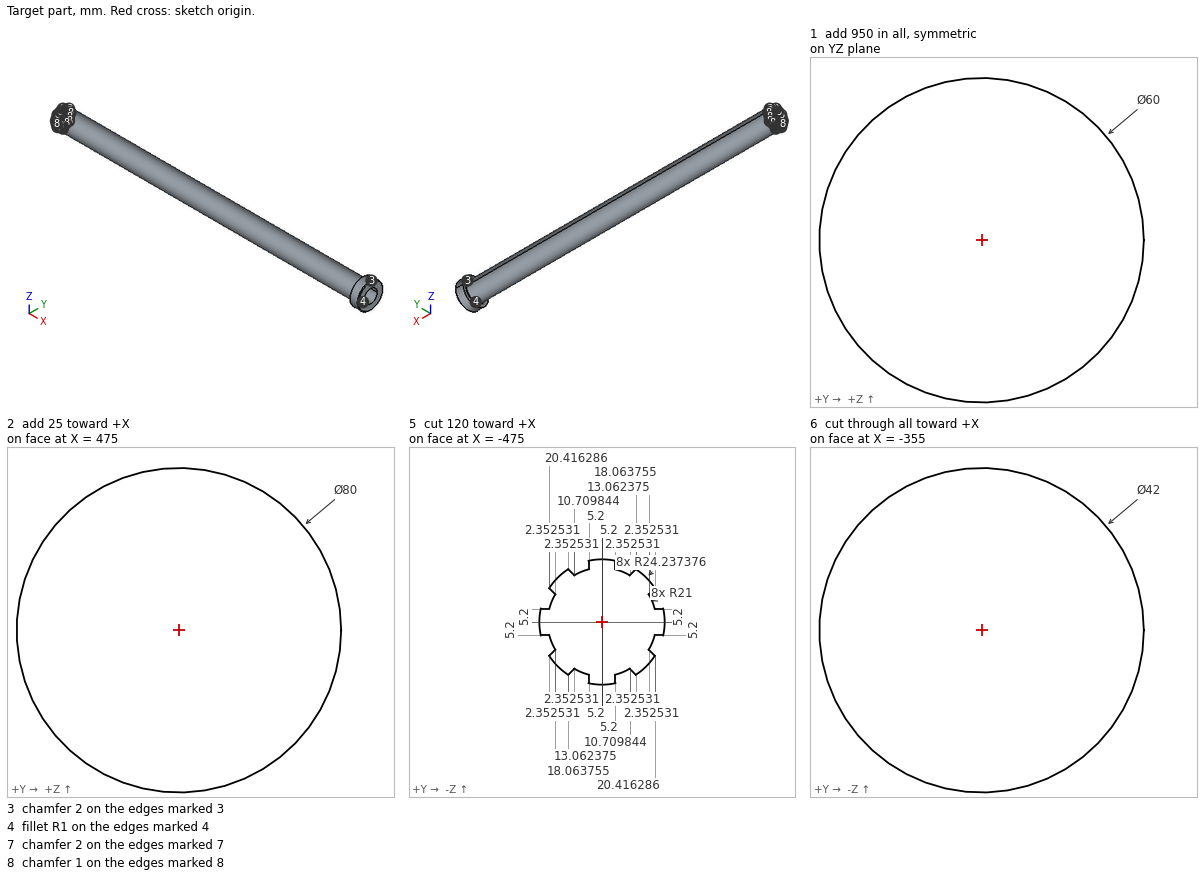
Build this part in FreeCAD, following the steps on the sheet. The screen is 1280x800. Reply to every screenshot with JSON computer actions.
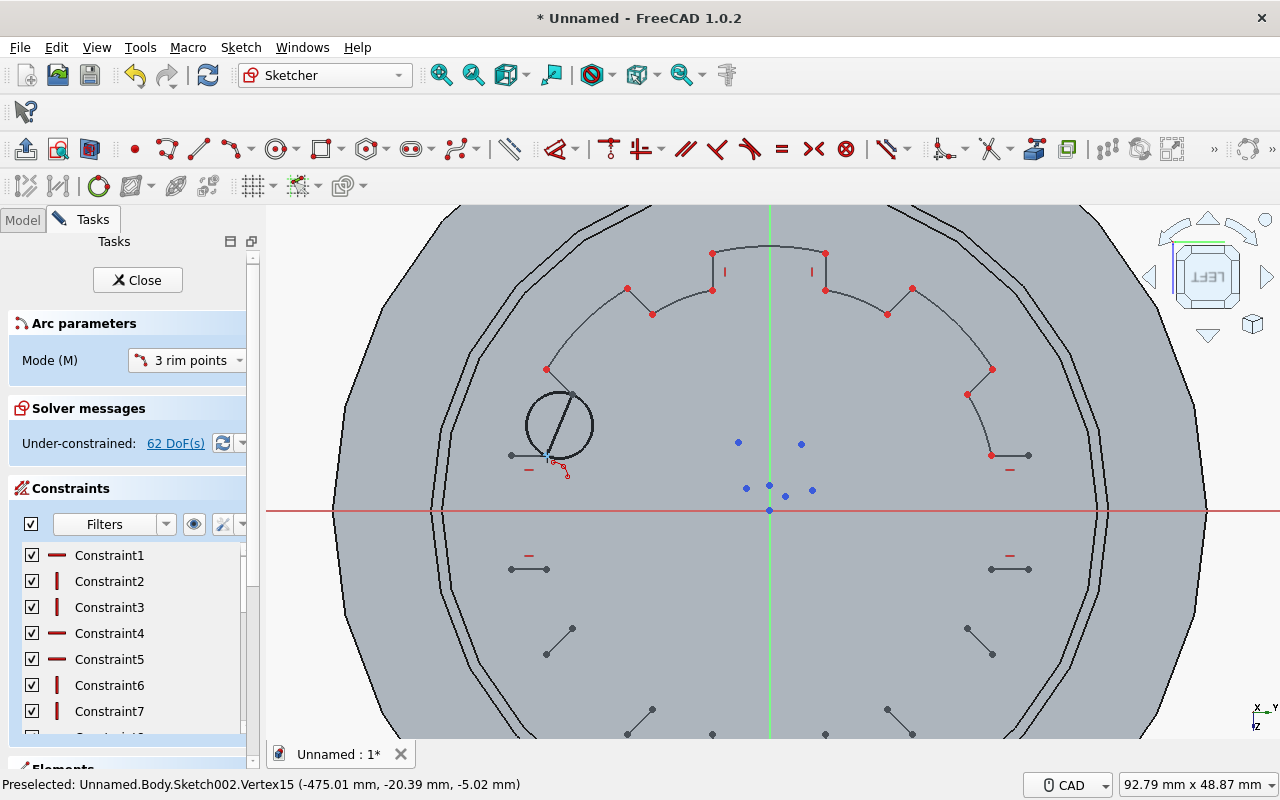
{"action": "scroll", "coordinate": [558, 423], "scroll_direction": "up", "scroll_amount": 10}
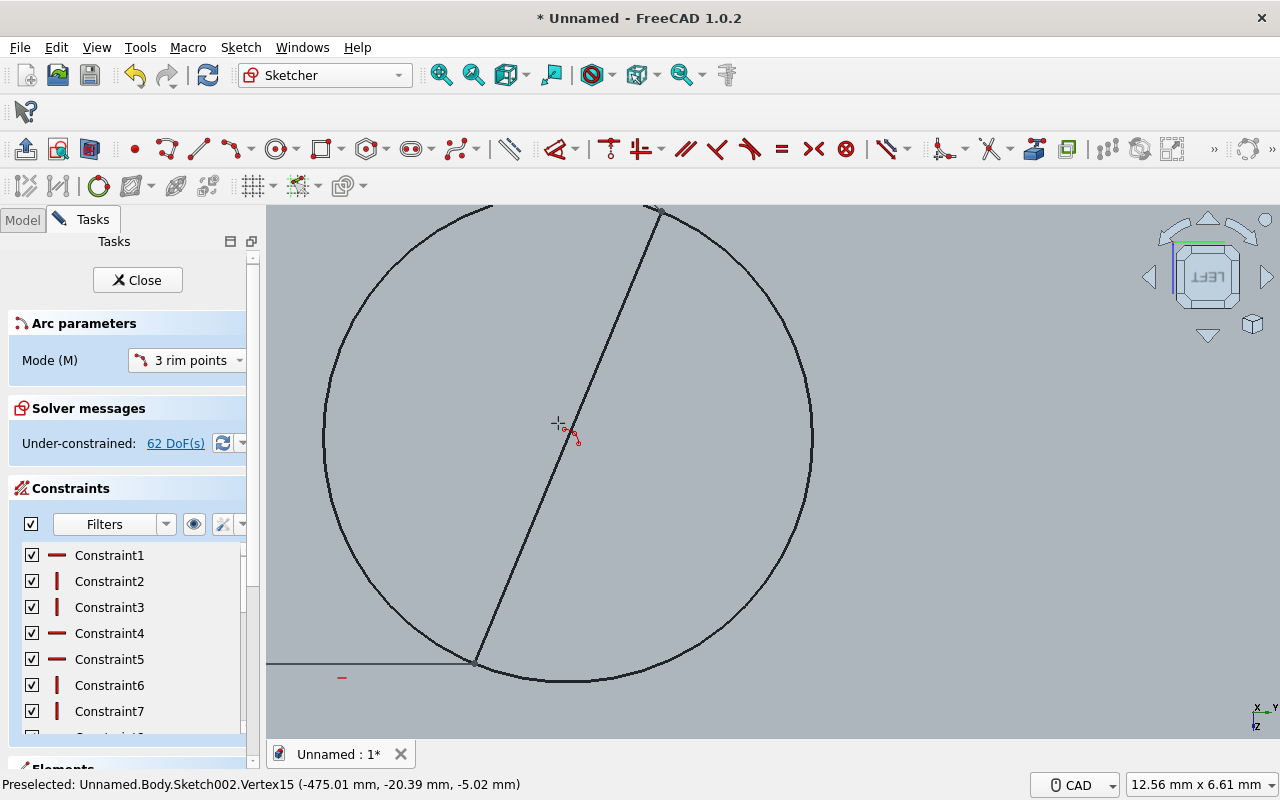
{"action": "left_click", "coordinate": [554, 420]}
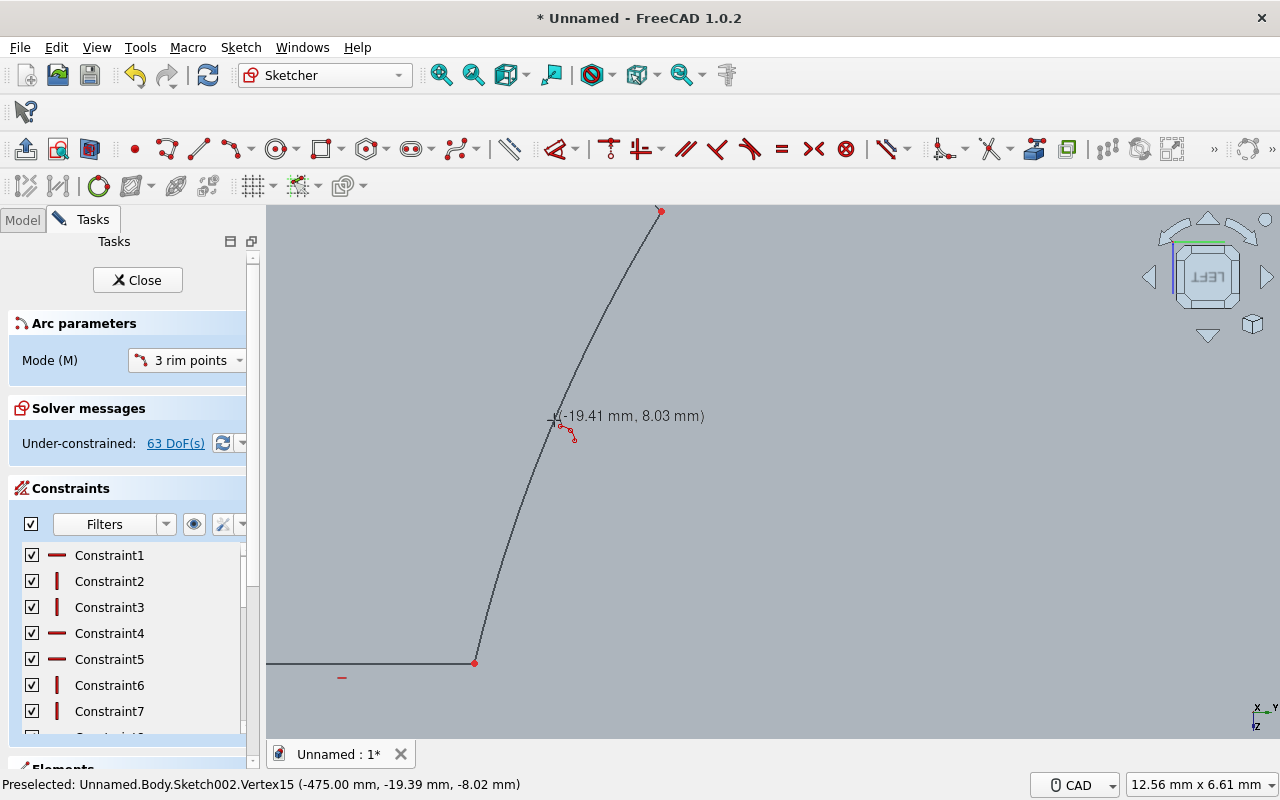
{"action": "scroll", "coordinate": [563, 412], "scroll_direction": "down", "scroll_amount": 12}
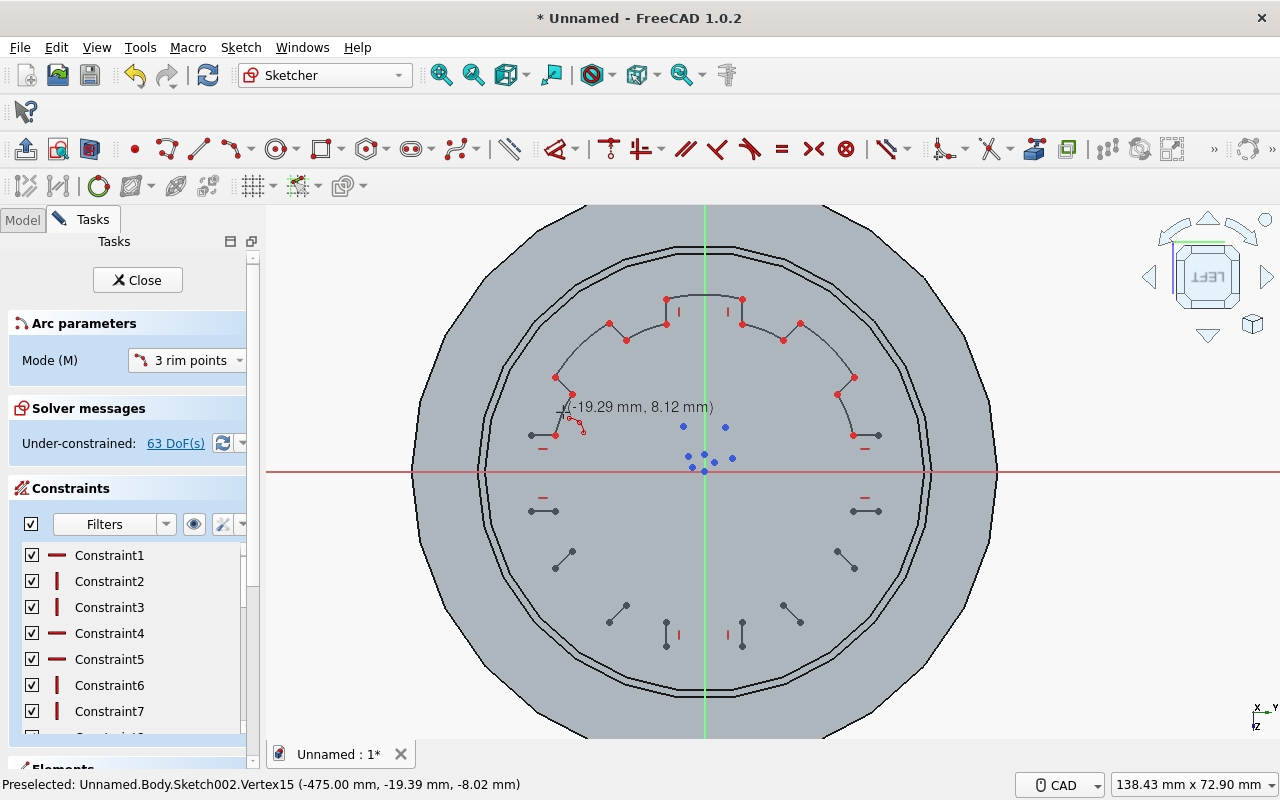
{"action": "scroll", "coordinate": [531, 434], "scroll_direction": "up", "scroll_amount": 2}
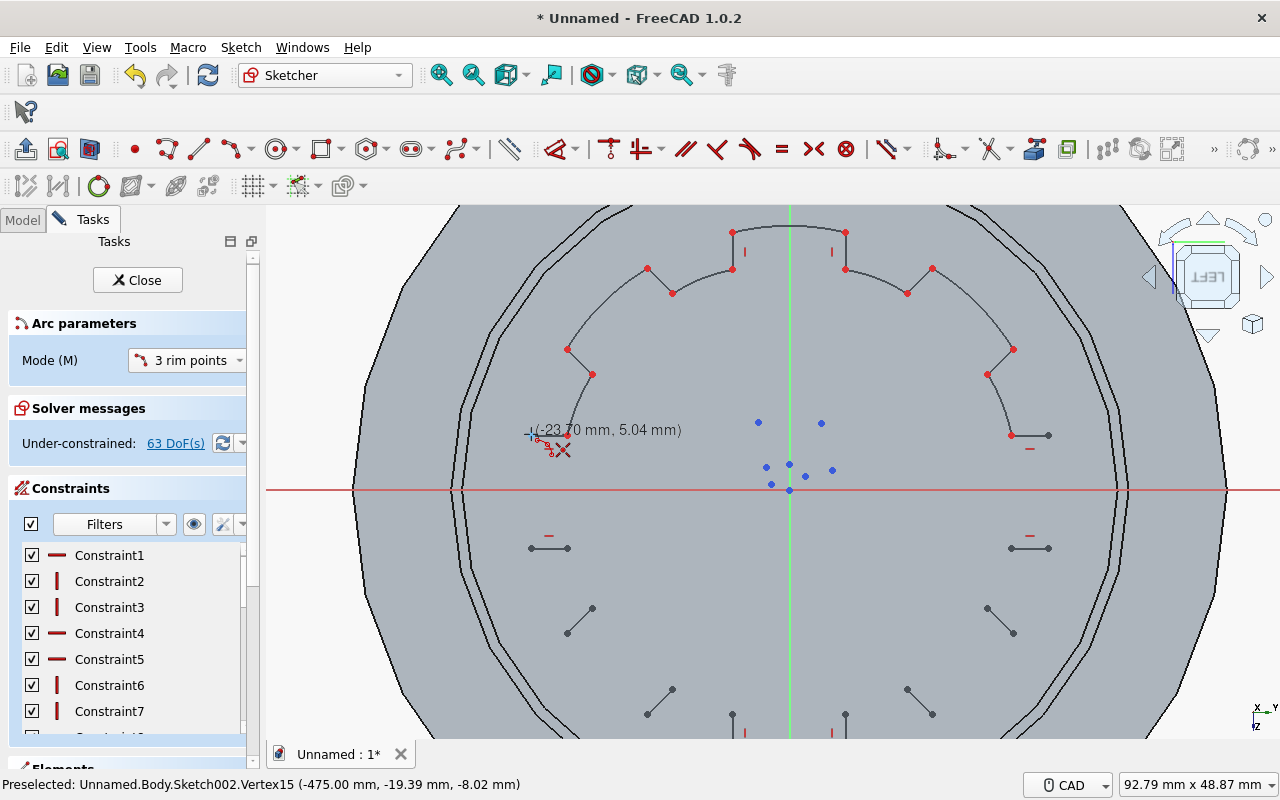
{"action": "left_click", "coordinate": [531, 436]}
{"action": "left_click", "coordinate": [531, 549]}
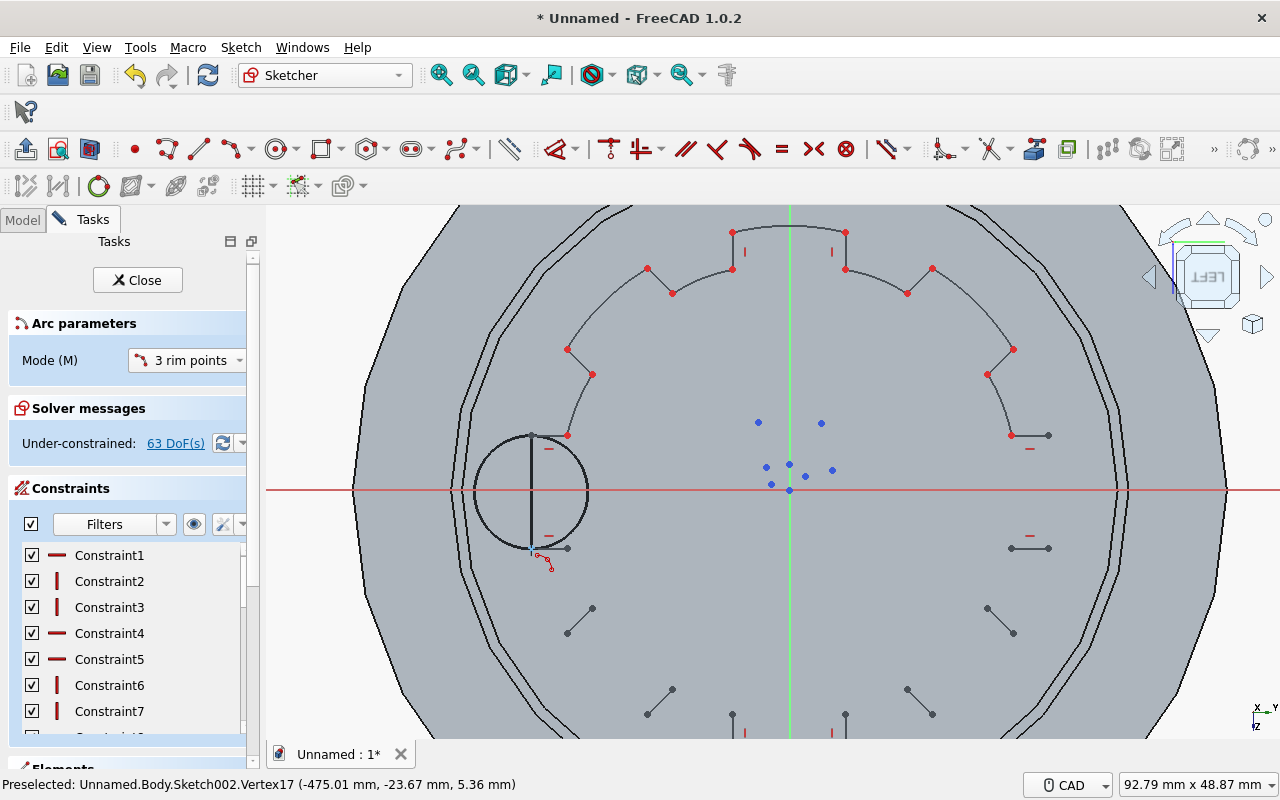
{"action": "scroll", "coordinate": [525, 479], "scroll_direction": "up", "scroll_amount": 5}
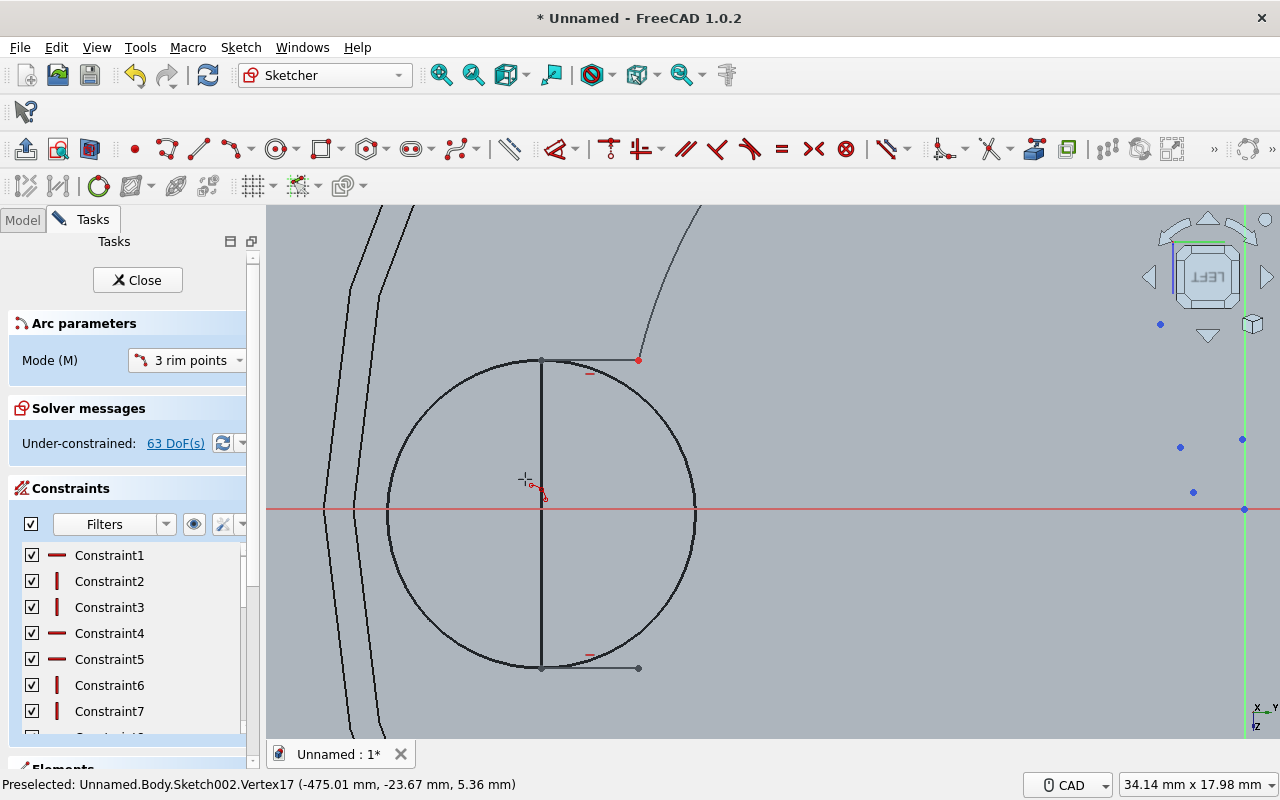
{"action": "left_click", "coordinate": [525, 478]}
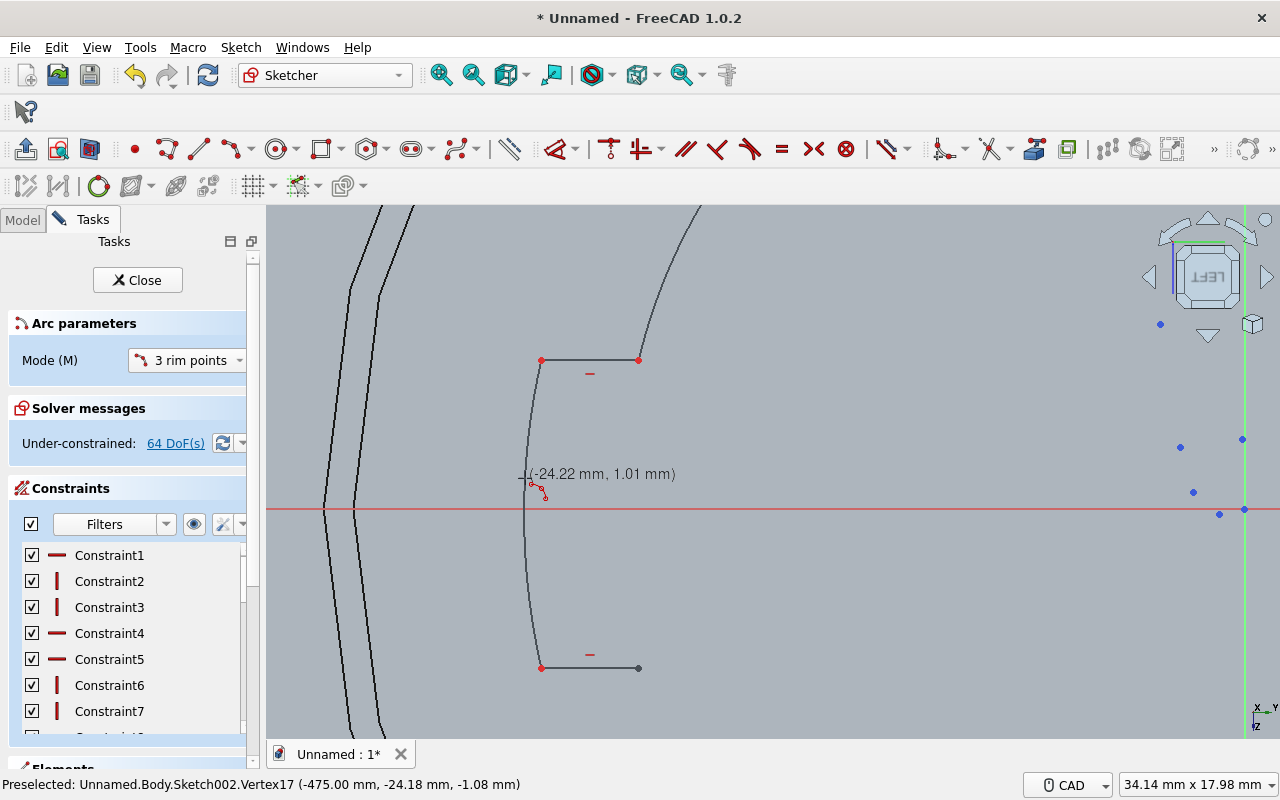
{"action": "scroll", "coordinate": [528, 460], "scroll_direction": "down", "scroll_amount": 7}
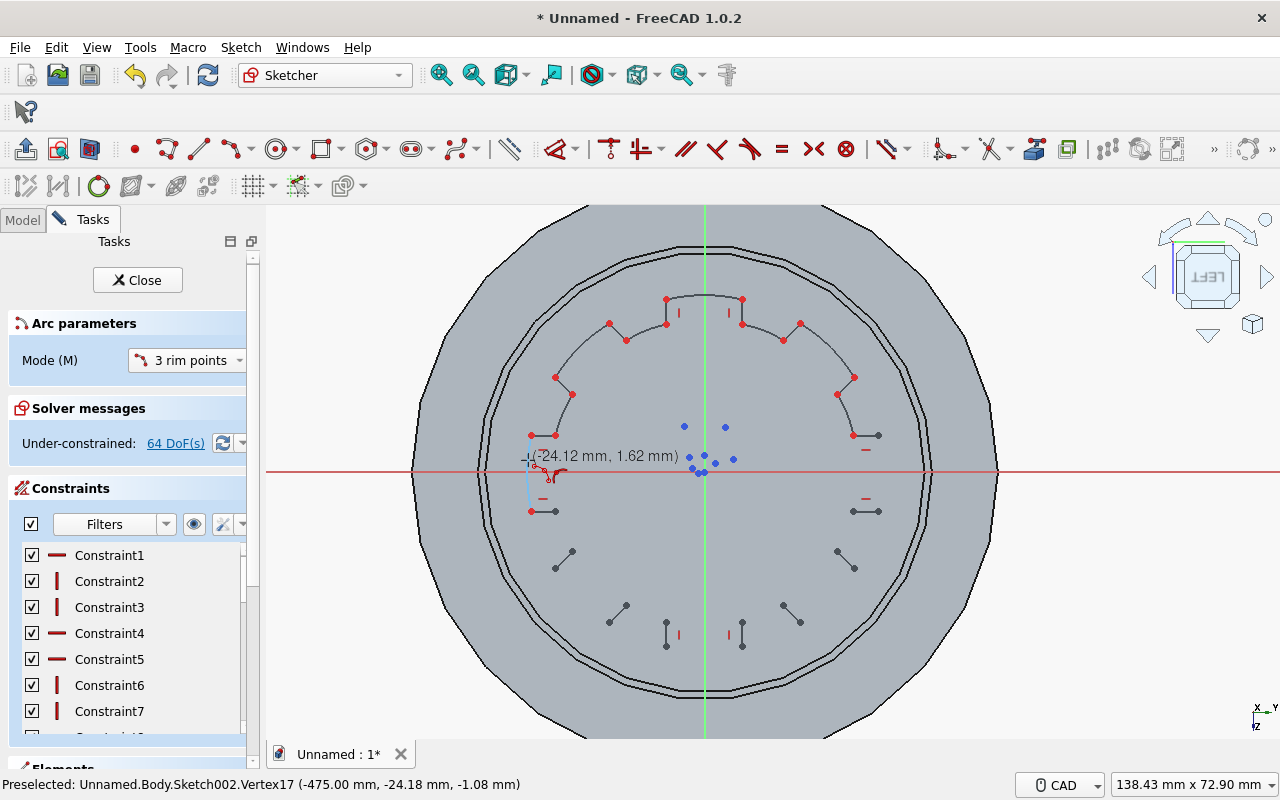
{"action": "scroll", "coordinate": [556, 511], "scroll_direction": "up", "scroll_amount": 2}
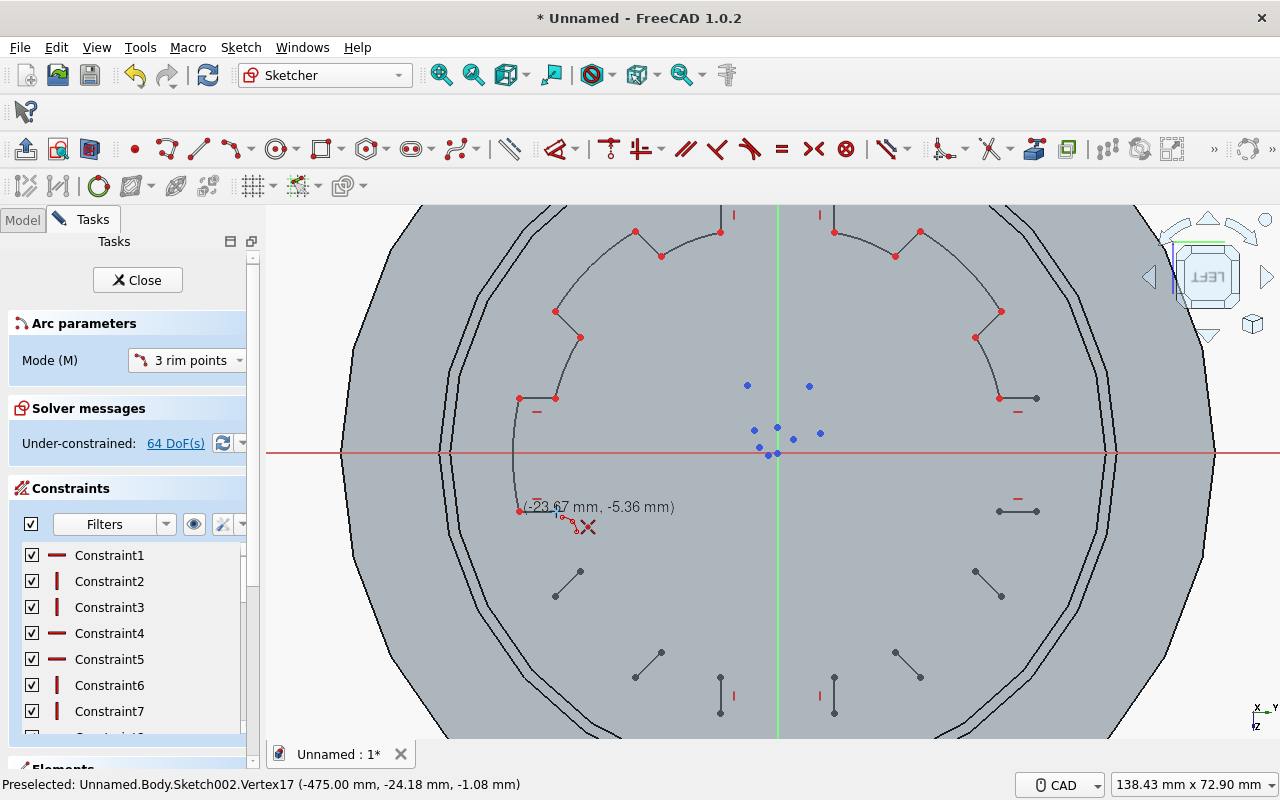
{"action": "left_click", "coordinate": [555, 512]}
{"action": "left_click", "coordinate": [580, 571]}